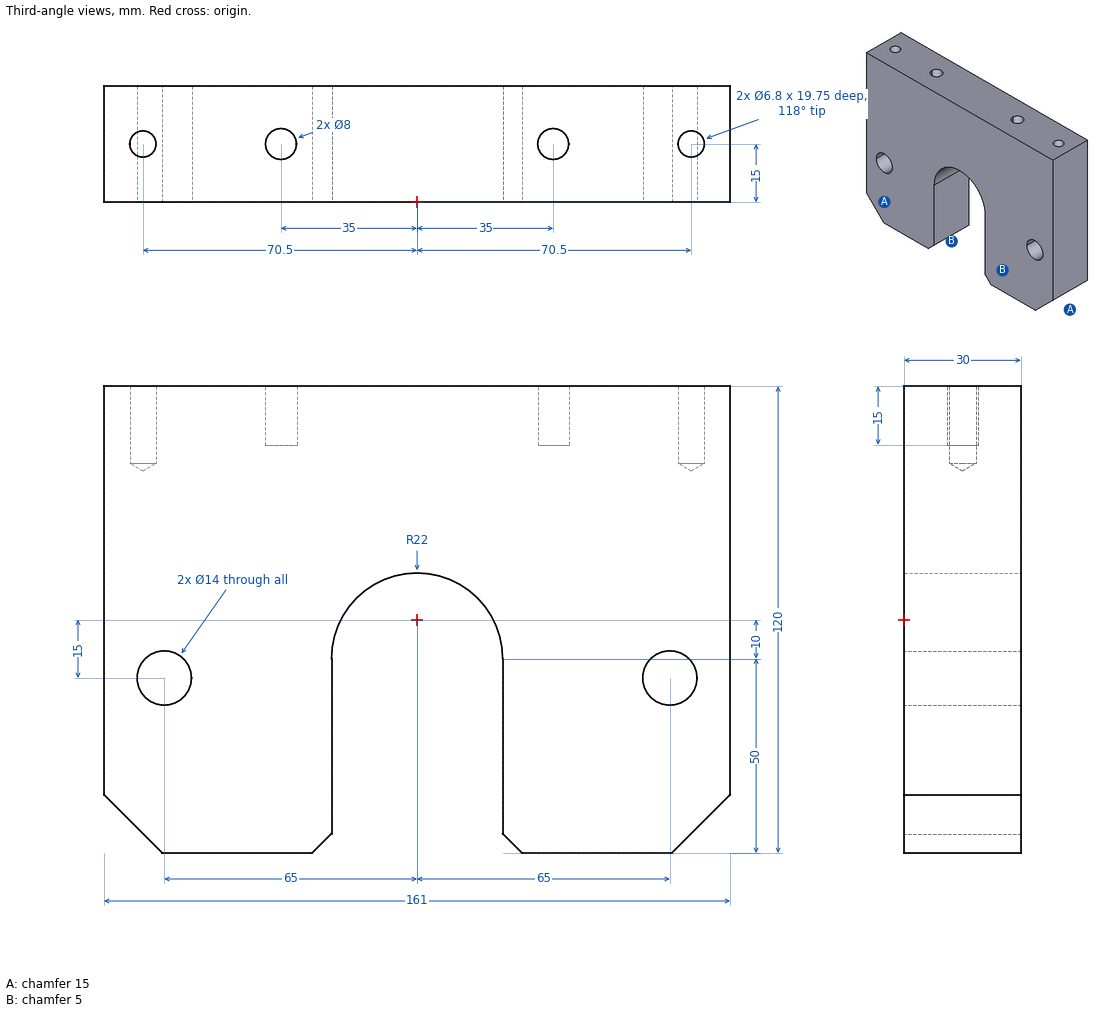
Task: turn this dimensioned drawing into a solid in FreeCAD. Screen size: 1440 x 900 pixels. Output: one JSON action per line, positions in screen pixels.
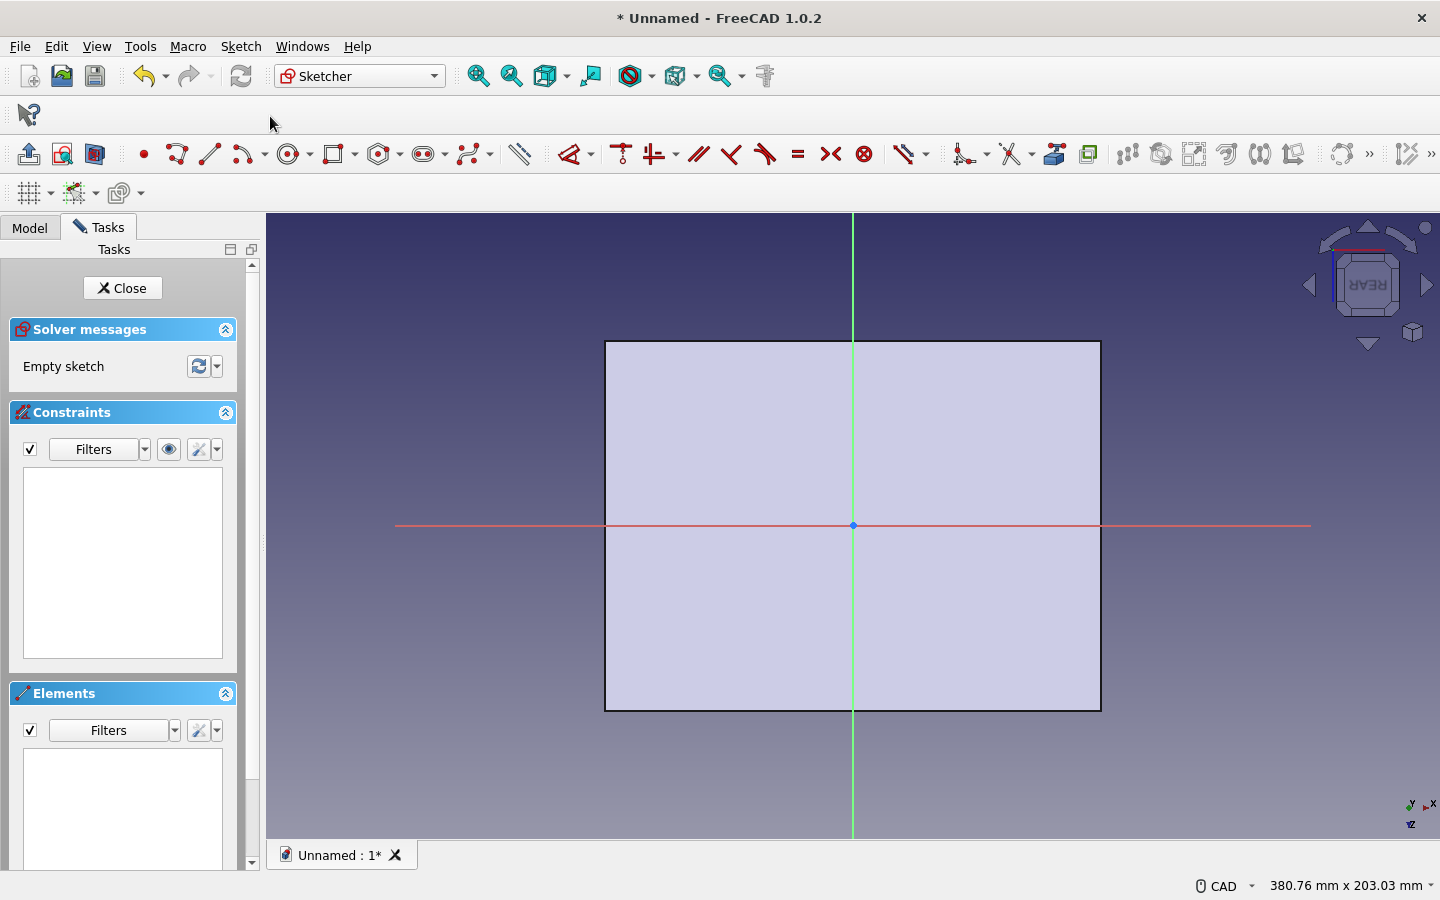
{"action": "scroll", "coordinate": [936, 362], "scroll_direction": "up", "scroll_amount": 3}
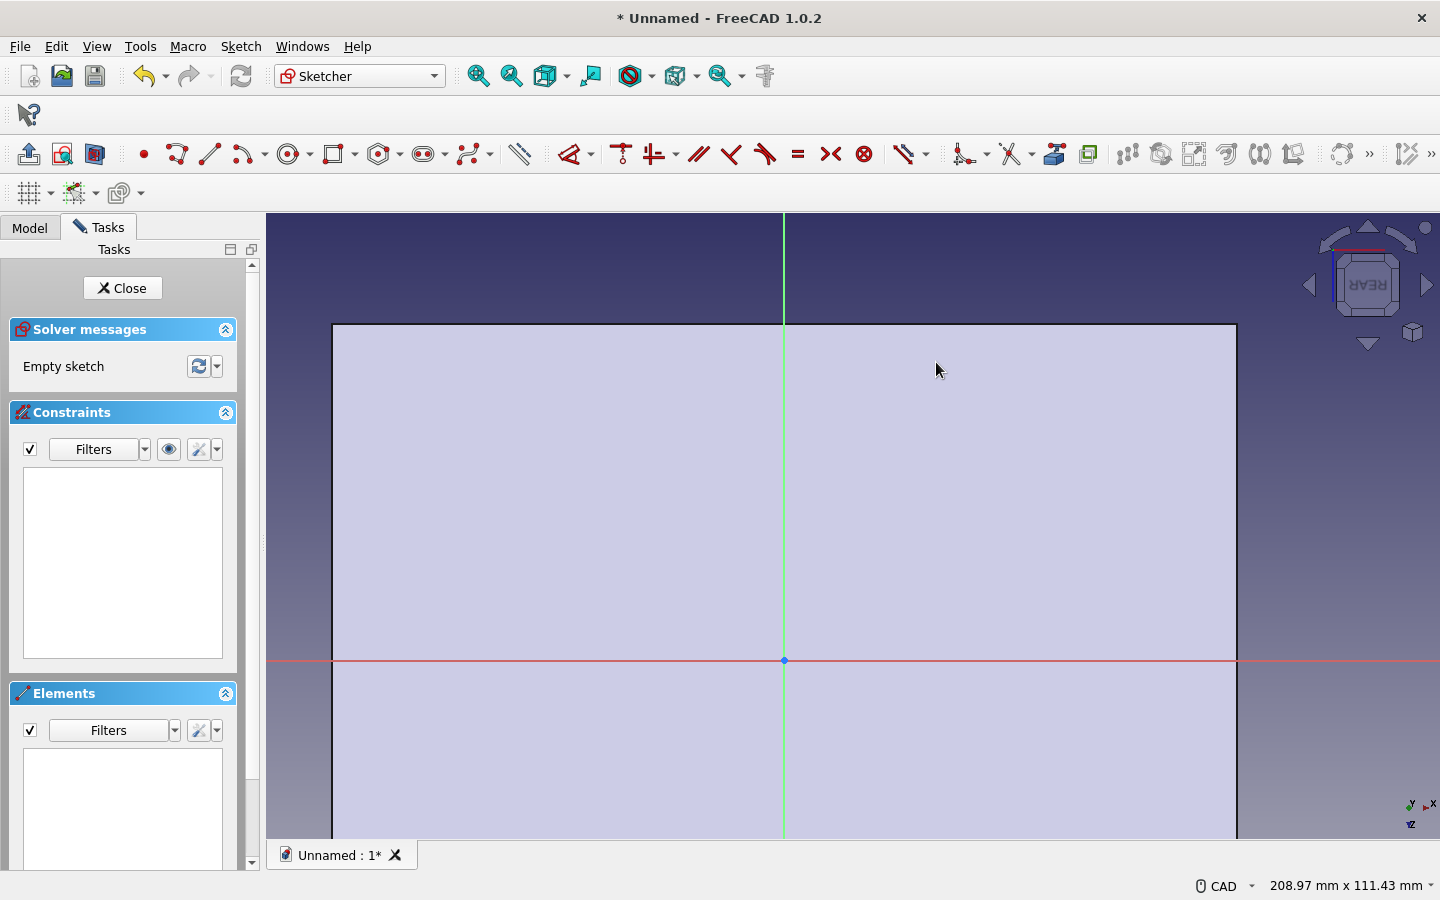
{"action": "key", "text": "g m"}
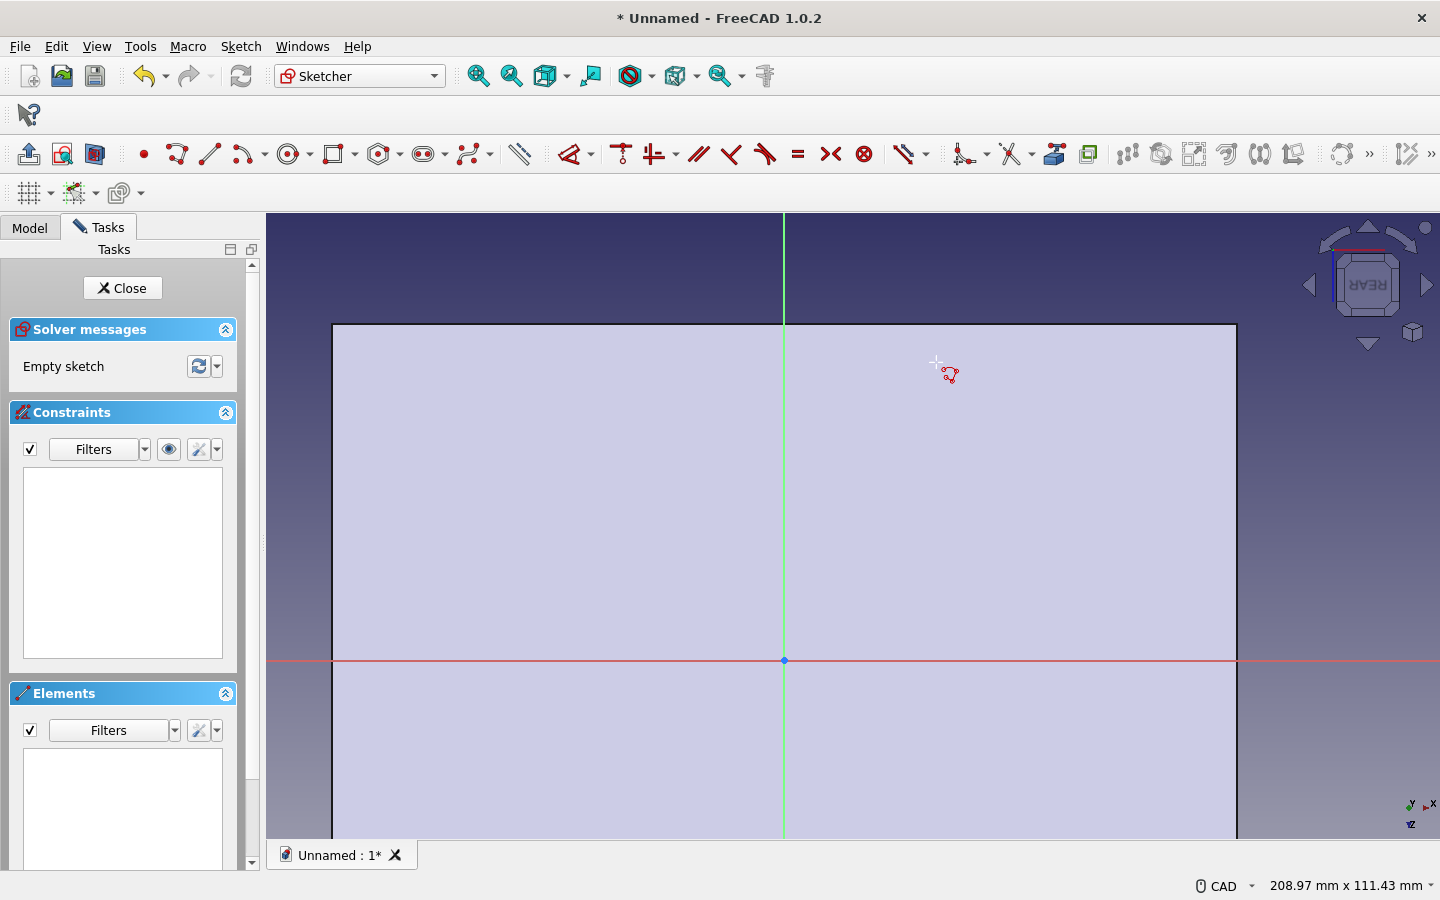
{"action": "left_click", "coordinate": [908, 604]}
{"action": "left_click", "coordinate": [908, 324]}
{"action": "left_click", "coordinate": [661, 324]}
{"action": "left_click", "coordinate": [661, 604]}
{"action": "right_click", "coordinate": [661, 604]}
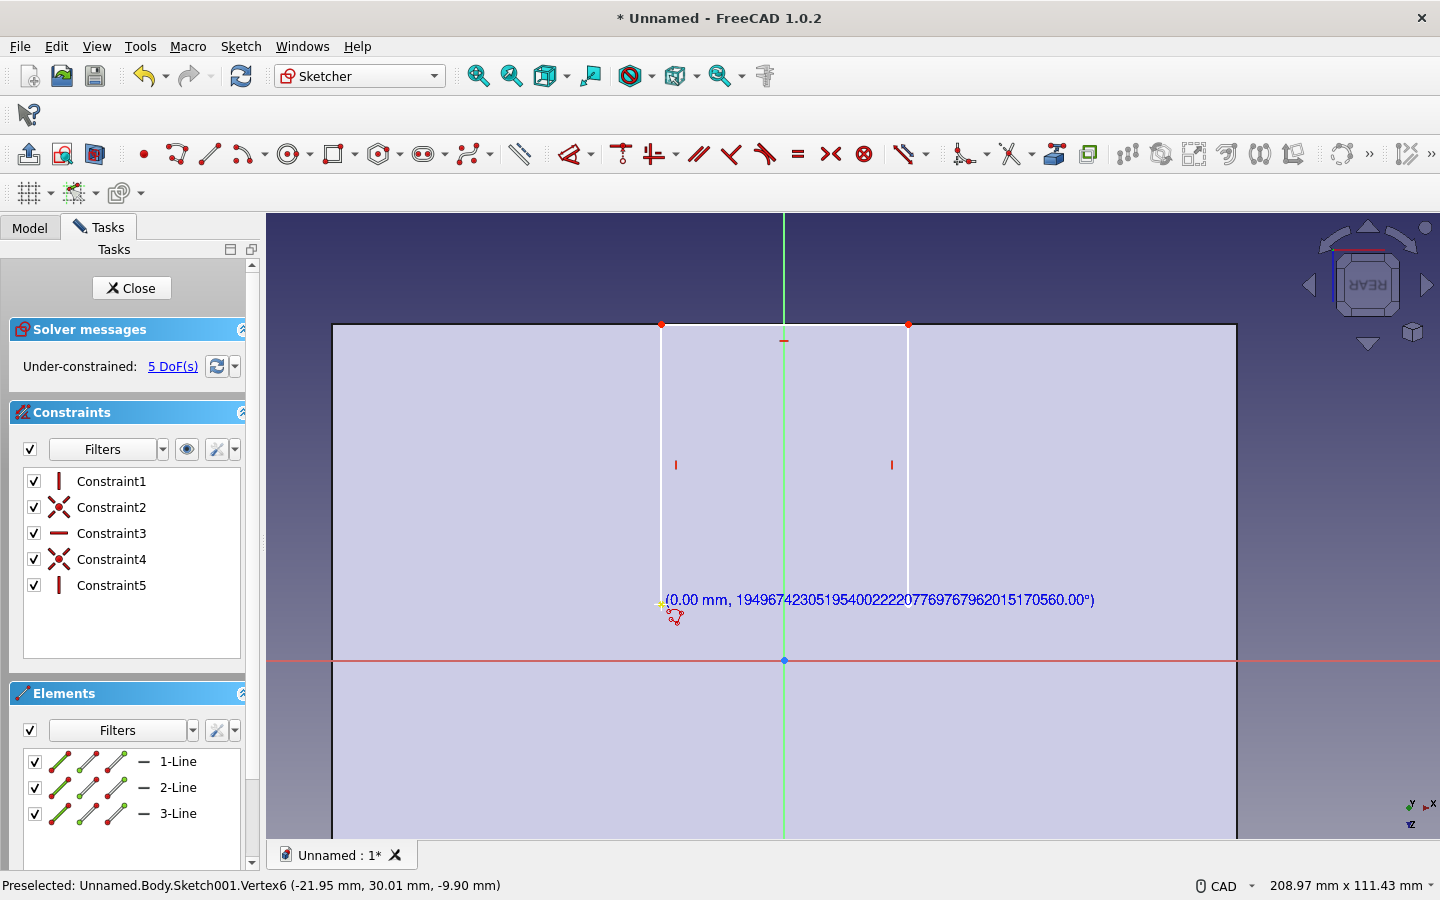
{"action": "left_click", "coordinate": [264, 154]}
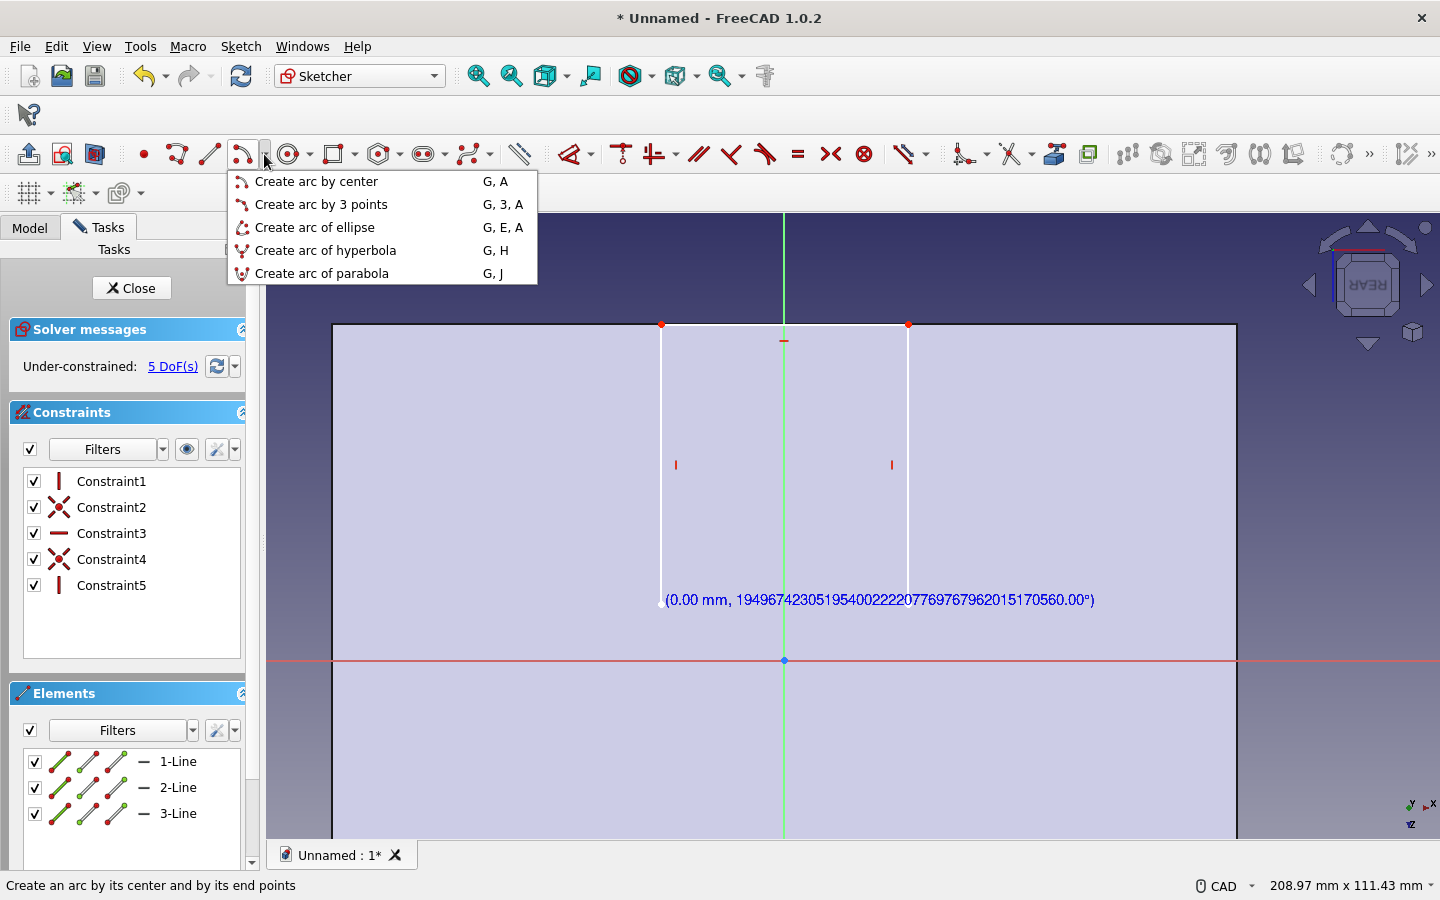
{"action": "left_click", "coordinate": [382, 204]}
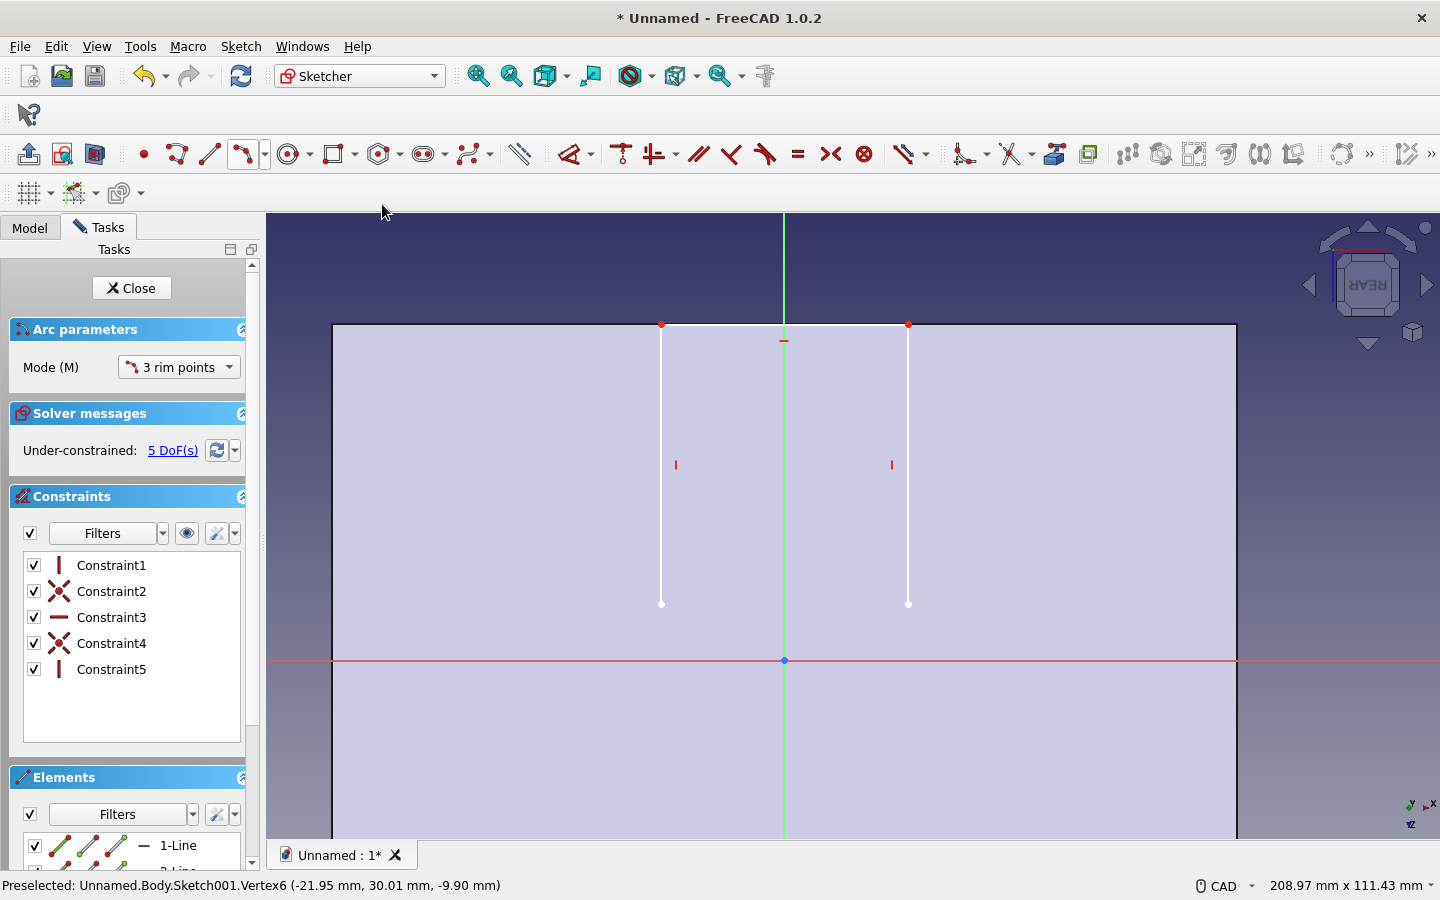
{"action": "left_click", "coordinate": [661, 605]}
{"action": "left_click", "coordinate": [908, 605]}
{"action": "left_click", "coordinate": [746, 722]}
{"action": "key", "text": "Escape"}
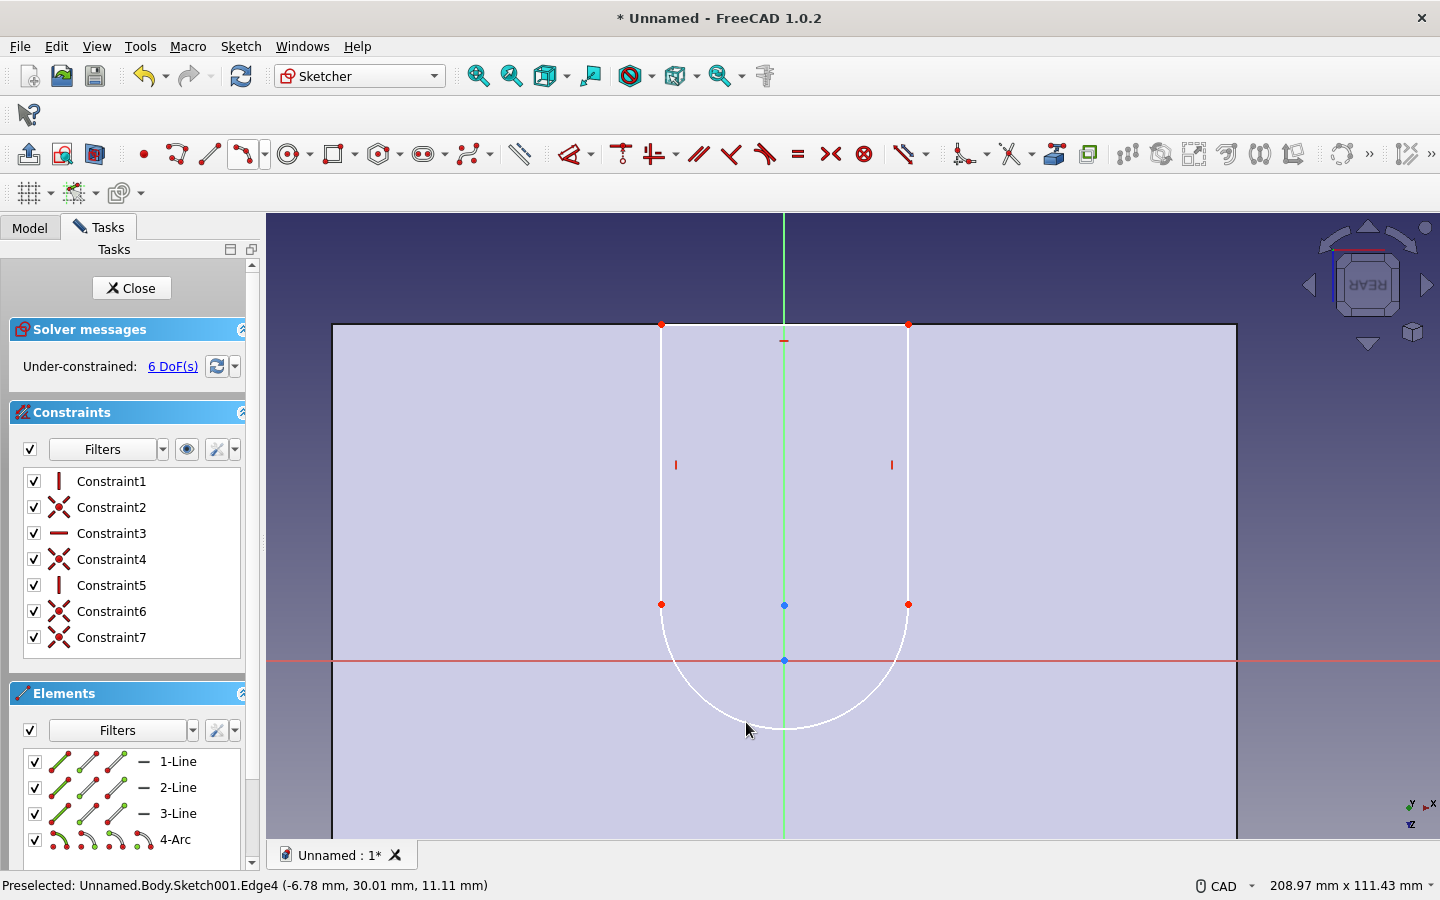
{"action": "left_click", "coordinate": [908, 521]}